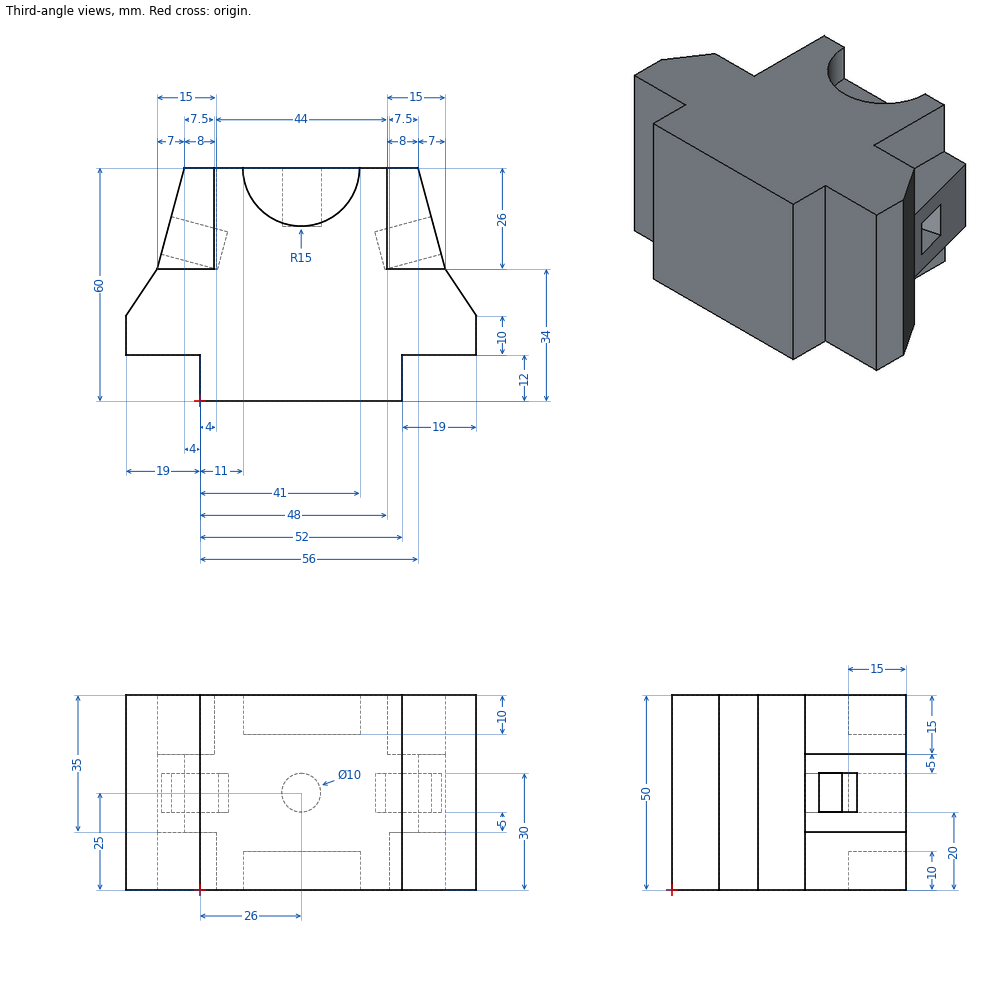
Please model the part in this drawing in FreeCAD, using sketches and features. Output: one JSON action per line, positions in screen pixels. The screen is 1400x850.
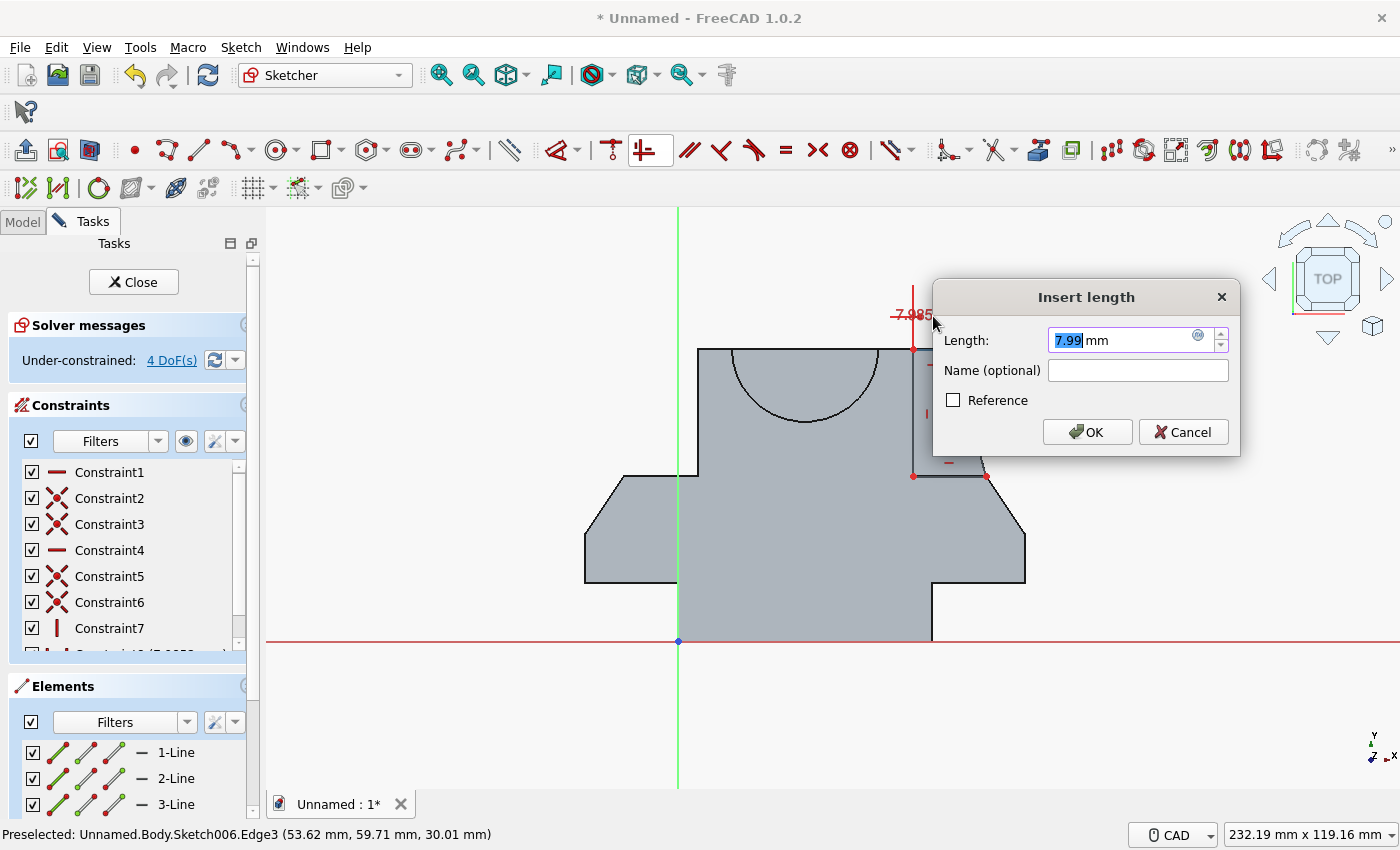
{"action": "type", "text": "8"}
{"action": "key", "text": "Return"}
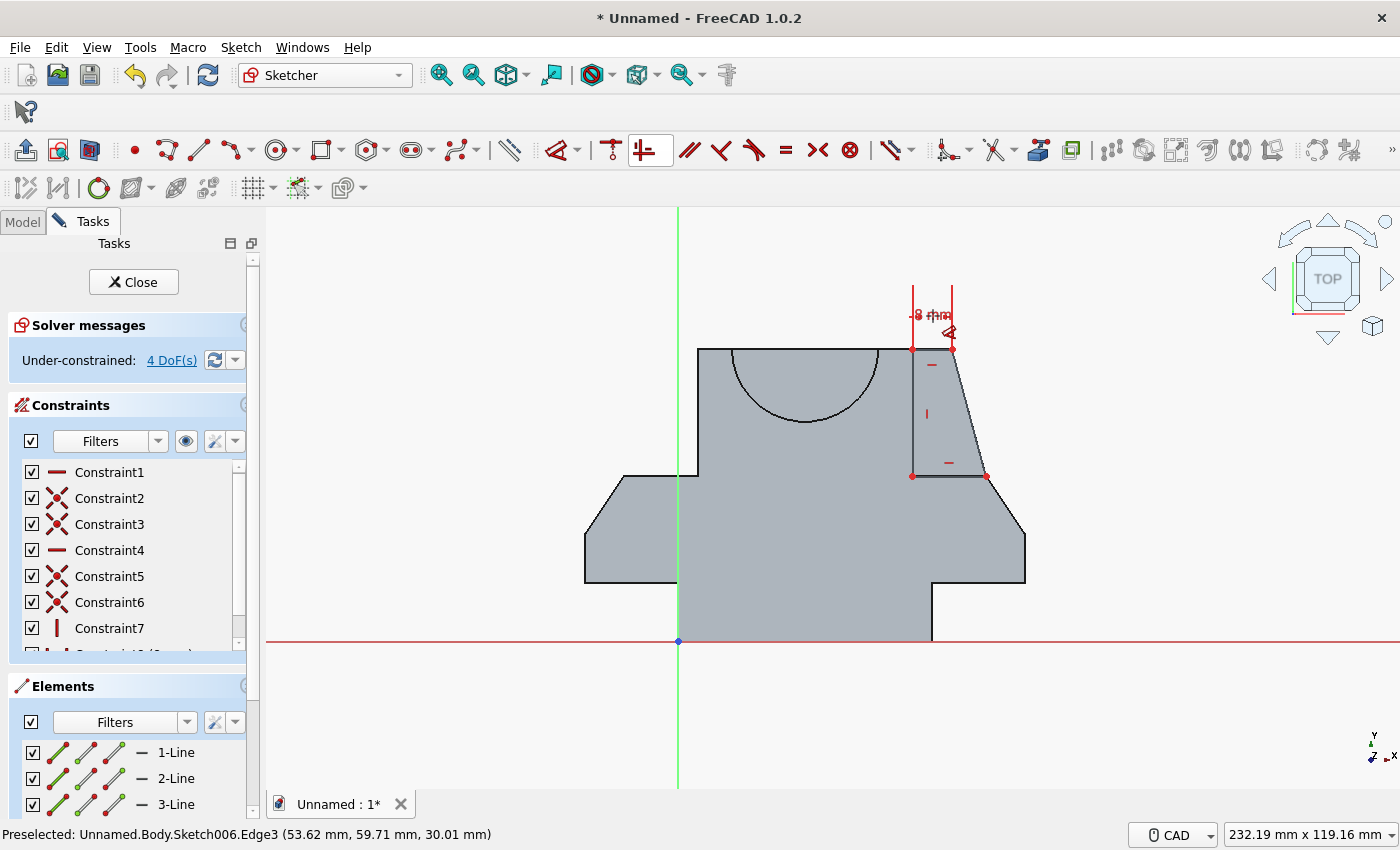
{"action": "left_click", "coordinate": [935, 477]}
{"action": "left_click", "coordinate": [949, 443]}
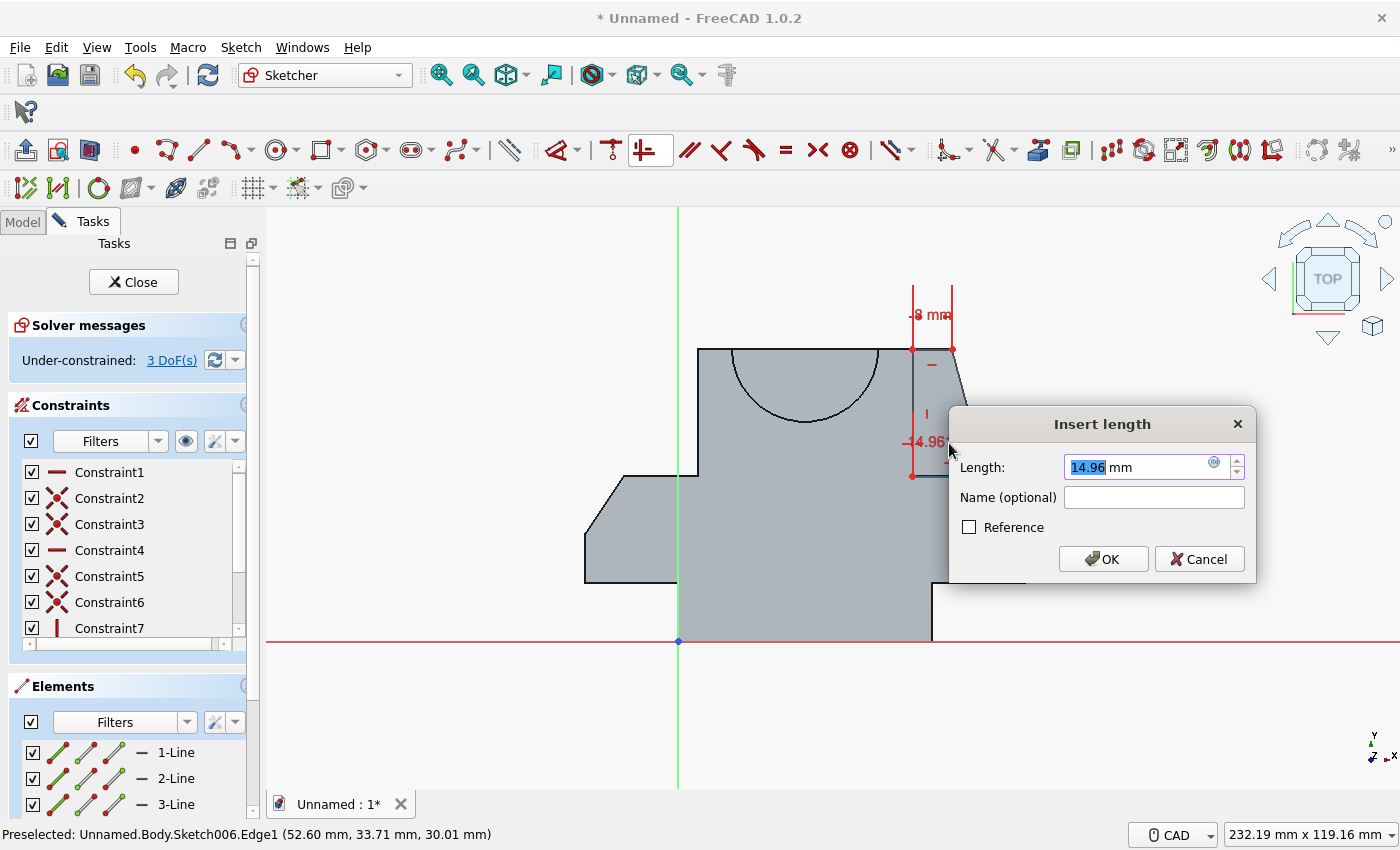
{"action": "type", "text": "15"}
{"action": "key", "text": "Return"}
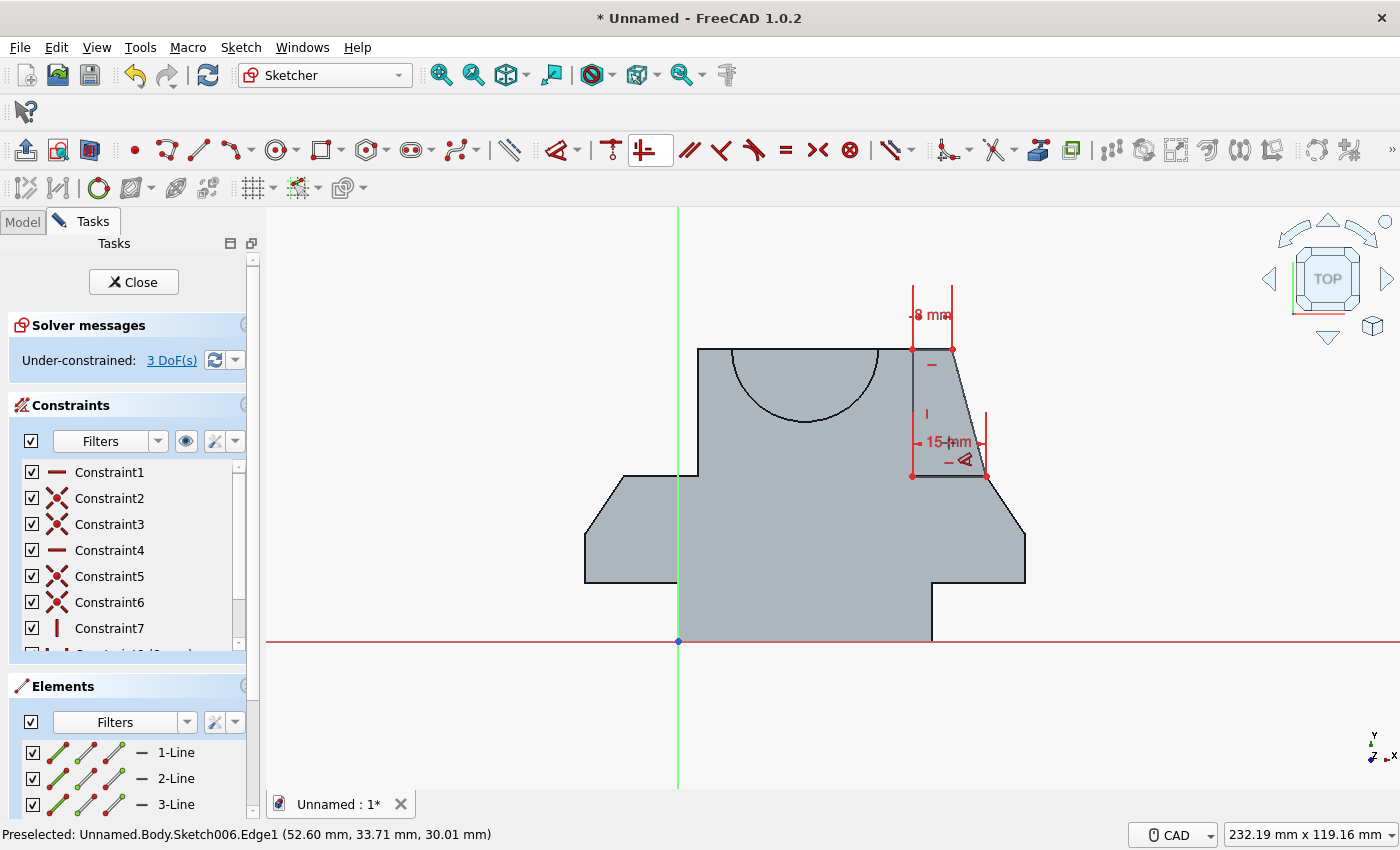
{"action": "left_click", "coordinate": [913, 388]}
{"action": "left_click", "coordinate": [947, 414]}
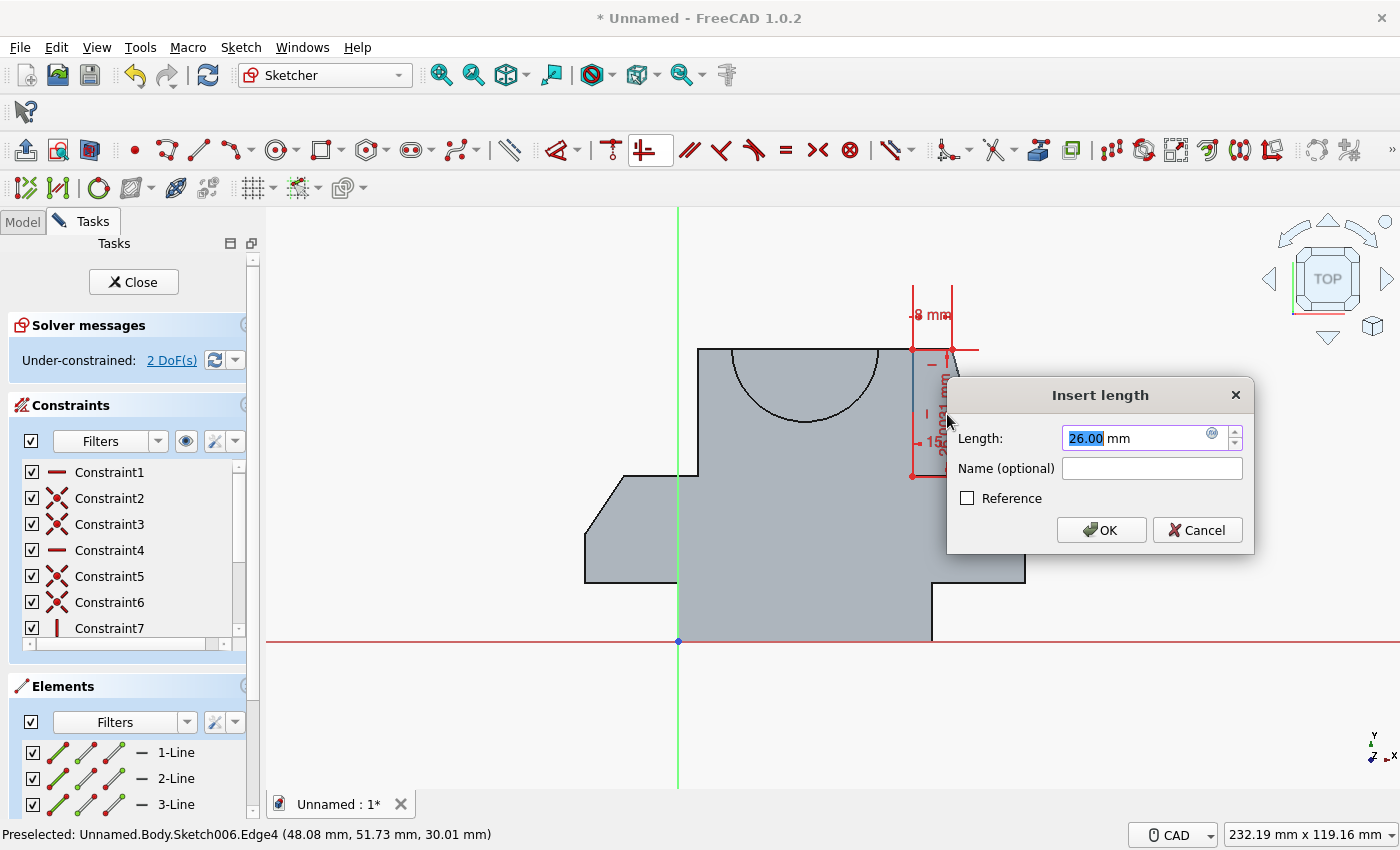
{"action": "type", "text": "26"}
{"action": "key", "text": "Return"}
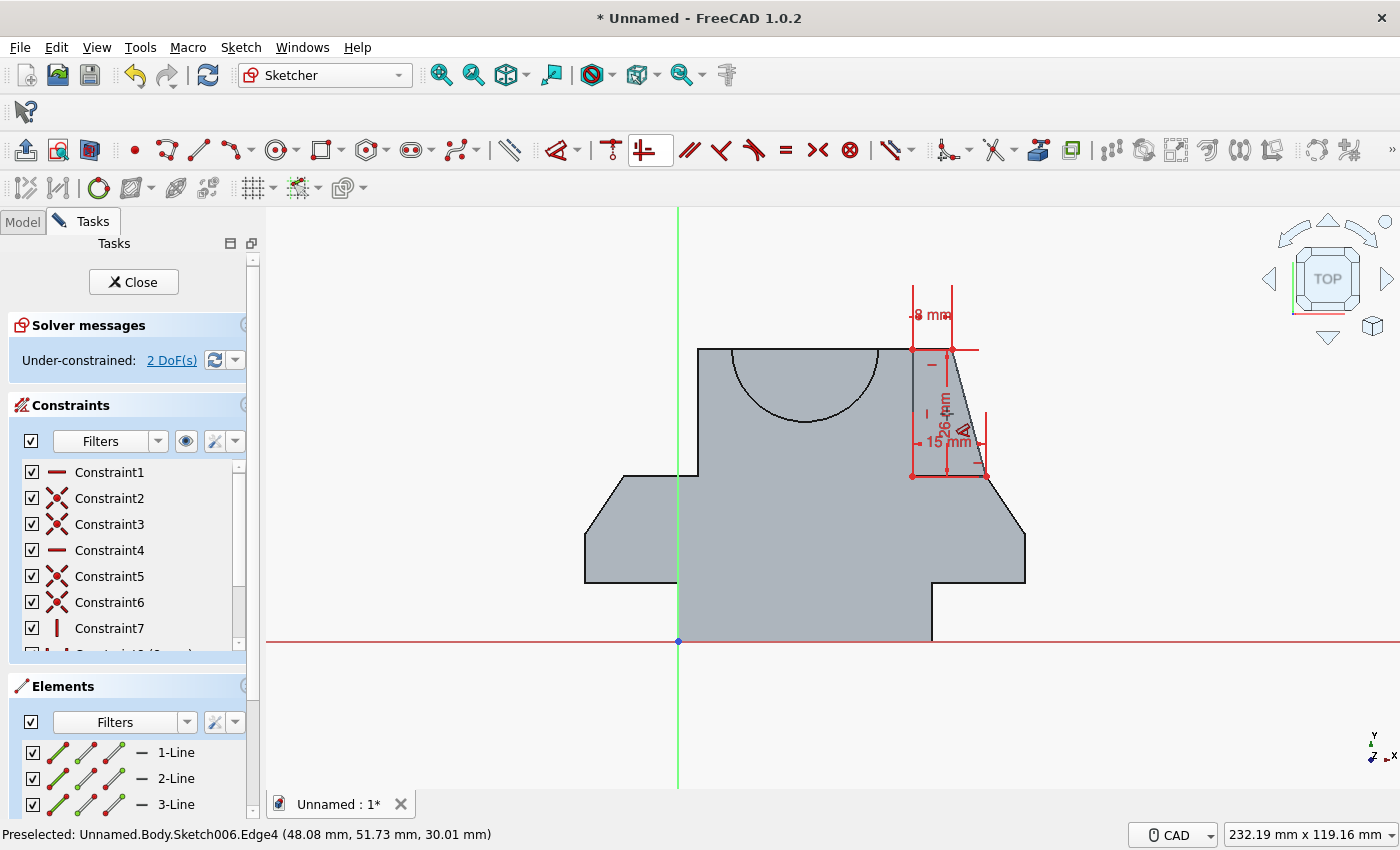
{"action": "left_click", "coordinate": [913, 477]}
{"action": "left_click", "coordinate": [796, 676]}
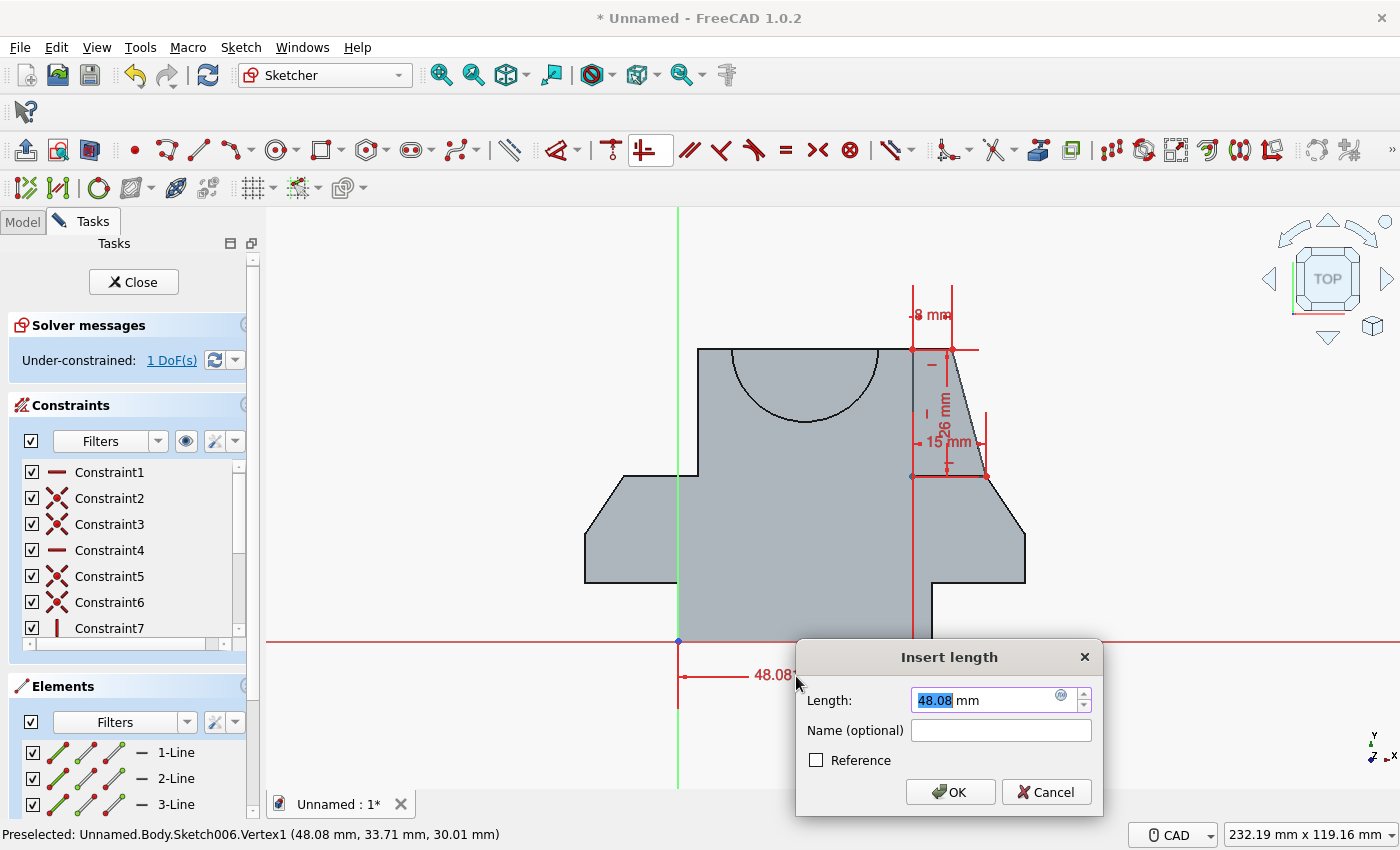
{"action": "type", "text": "48"}
{"action": "key", "text": "Return"}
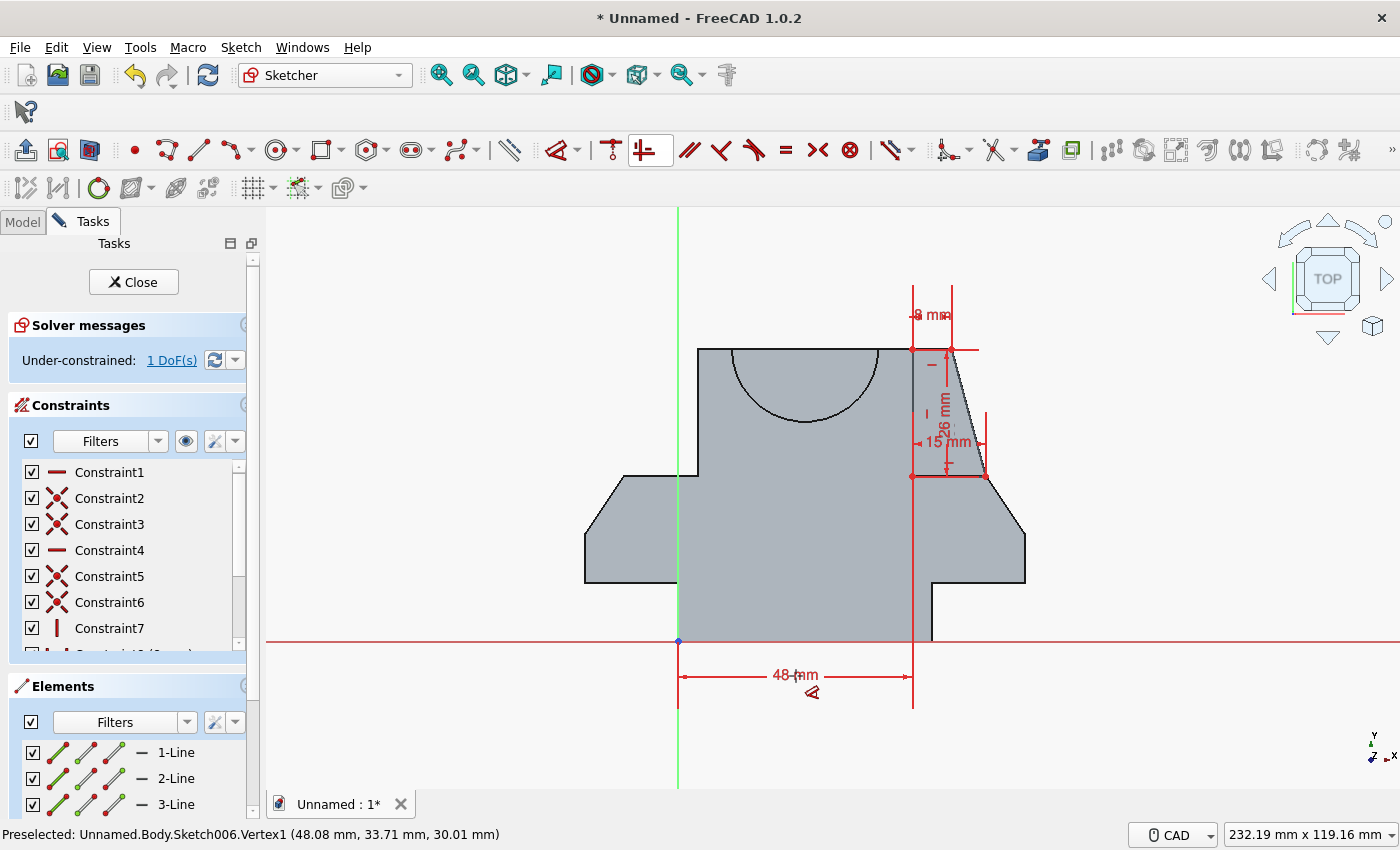
{"action": "left_click", "coordinate": [913, 477]}
{"action": "left_click", "coordinate": [644, 559]}